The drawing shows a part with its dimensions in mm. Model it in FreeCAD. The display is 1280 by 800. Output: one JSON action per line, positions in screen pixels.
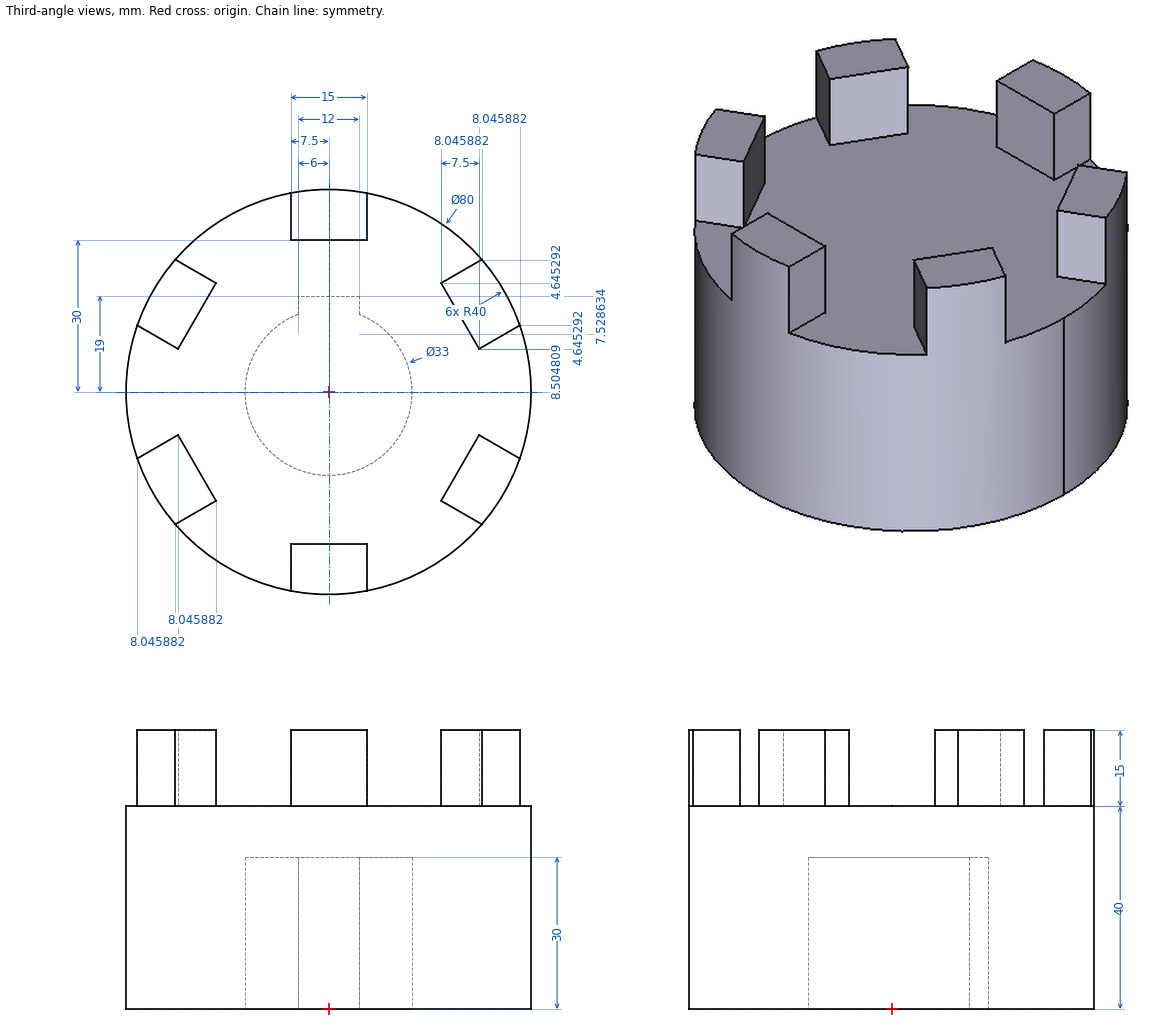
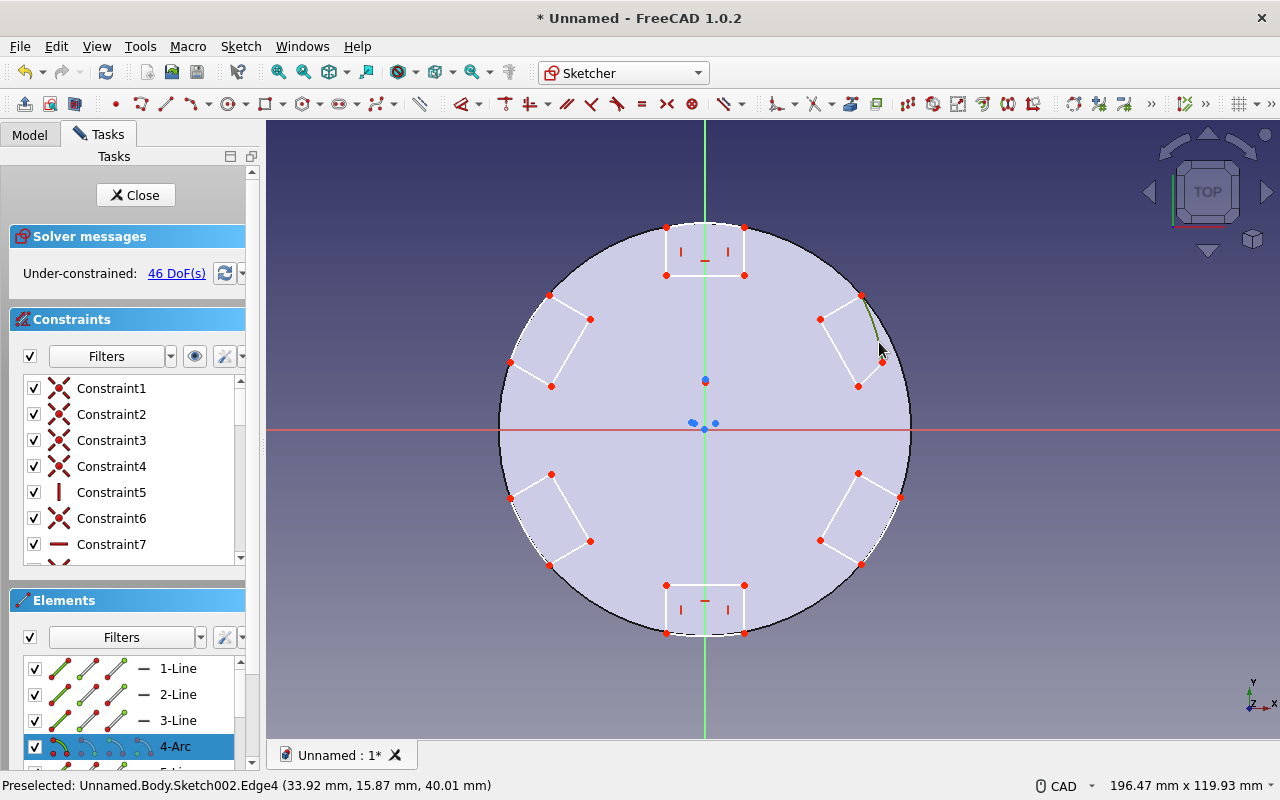
{"action": "left_click", "coordinate": [875, 546]}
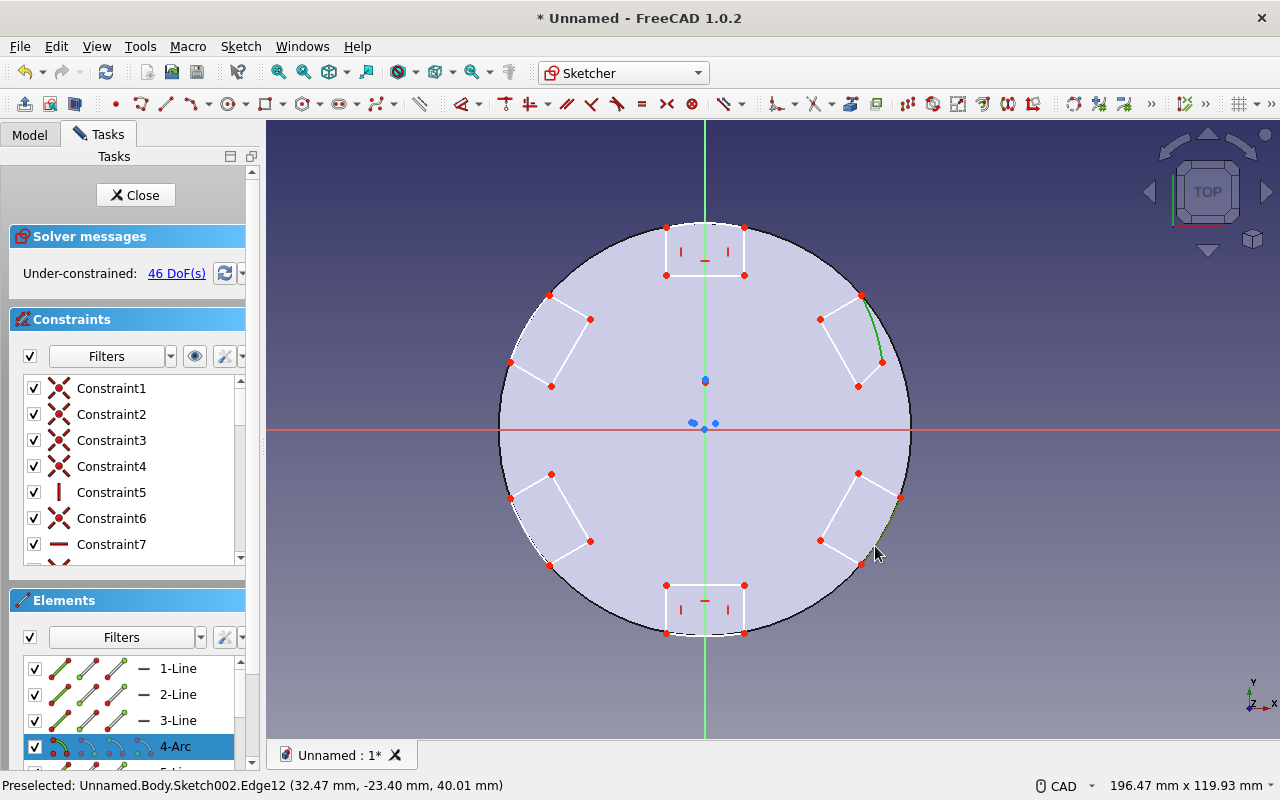
{"action": "key", "text": "c"}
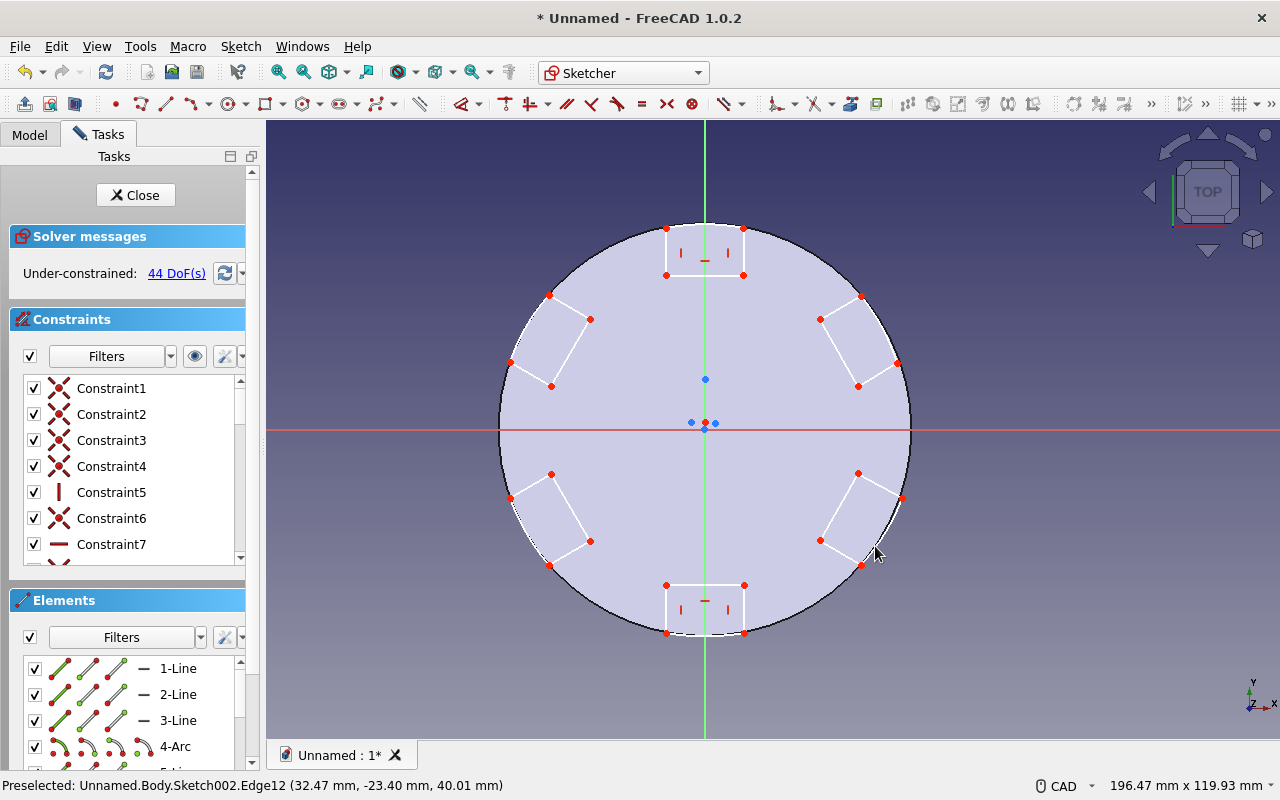
{"action": "left_click", "coordinate": [889, 342]}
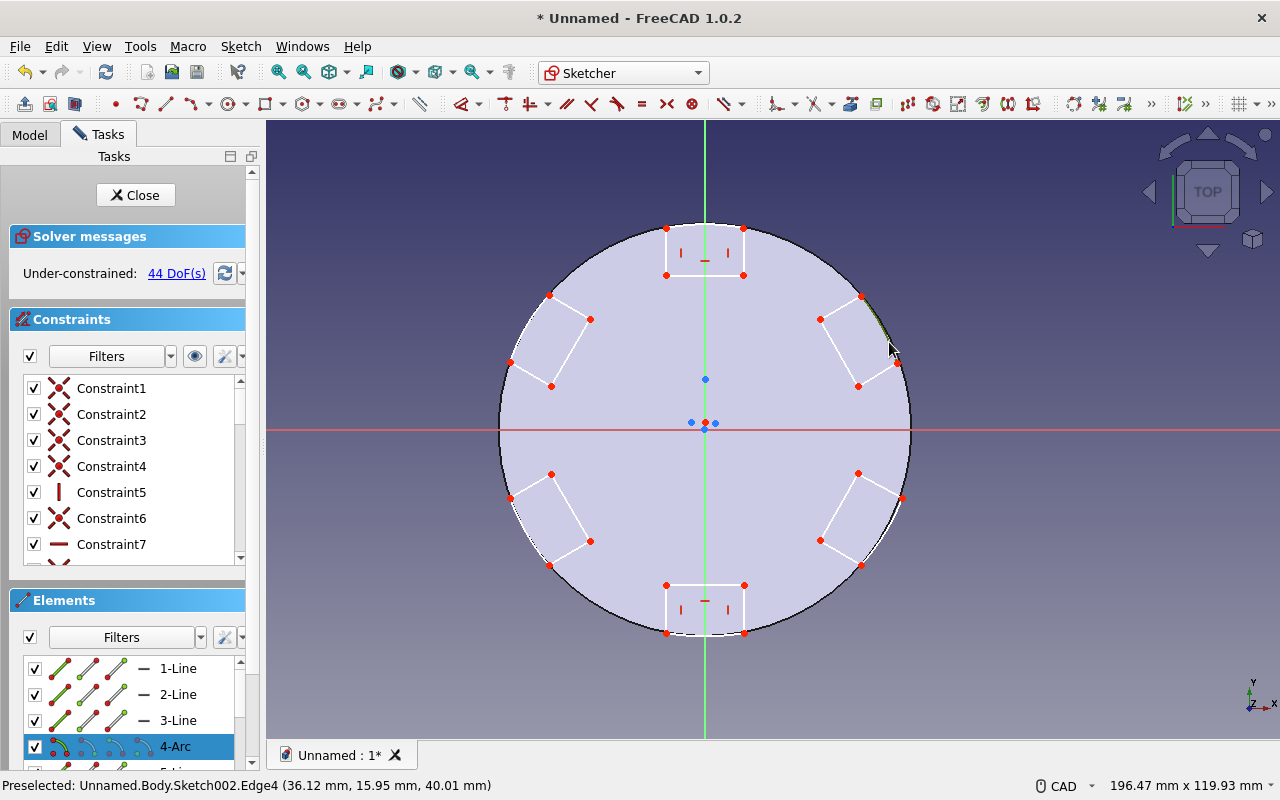
{"action": "left_click", "coordinate": [689, 636]}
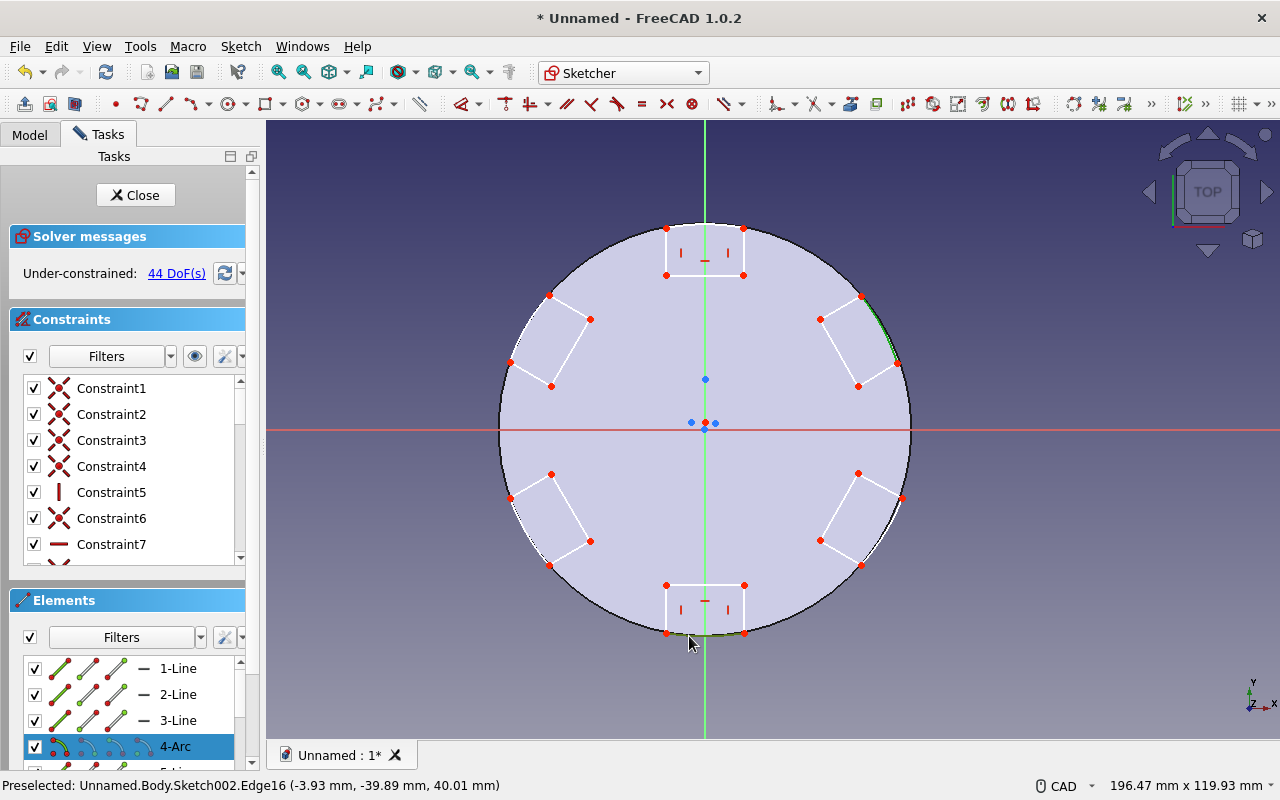
{"action": "key", "text": "c"}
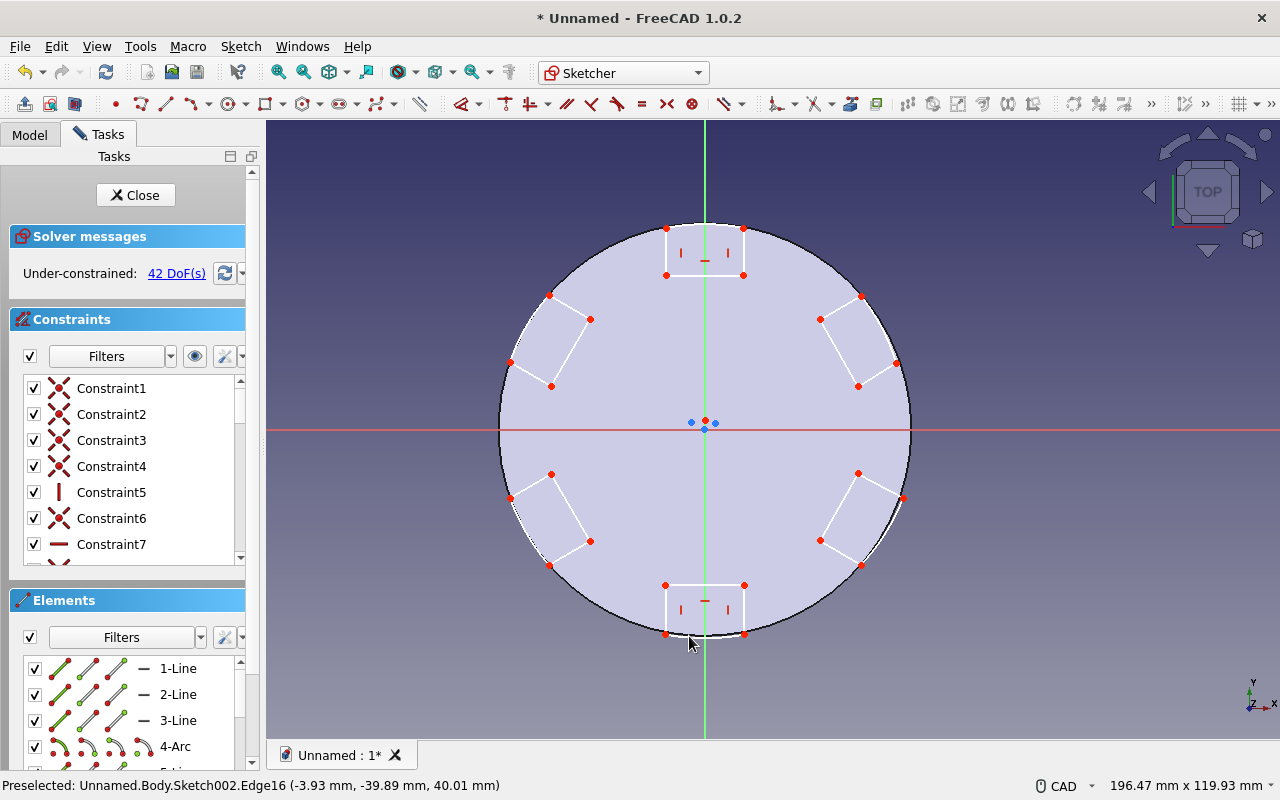
{"action": "left_click", "coordinate": [888, 342]}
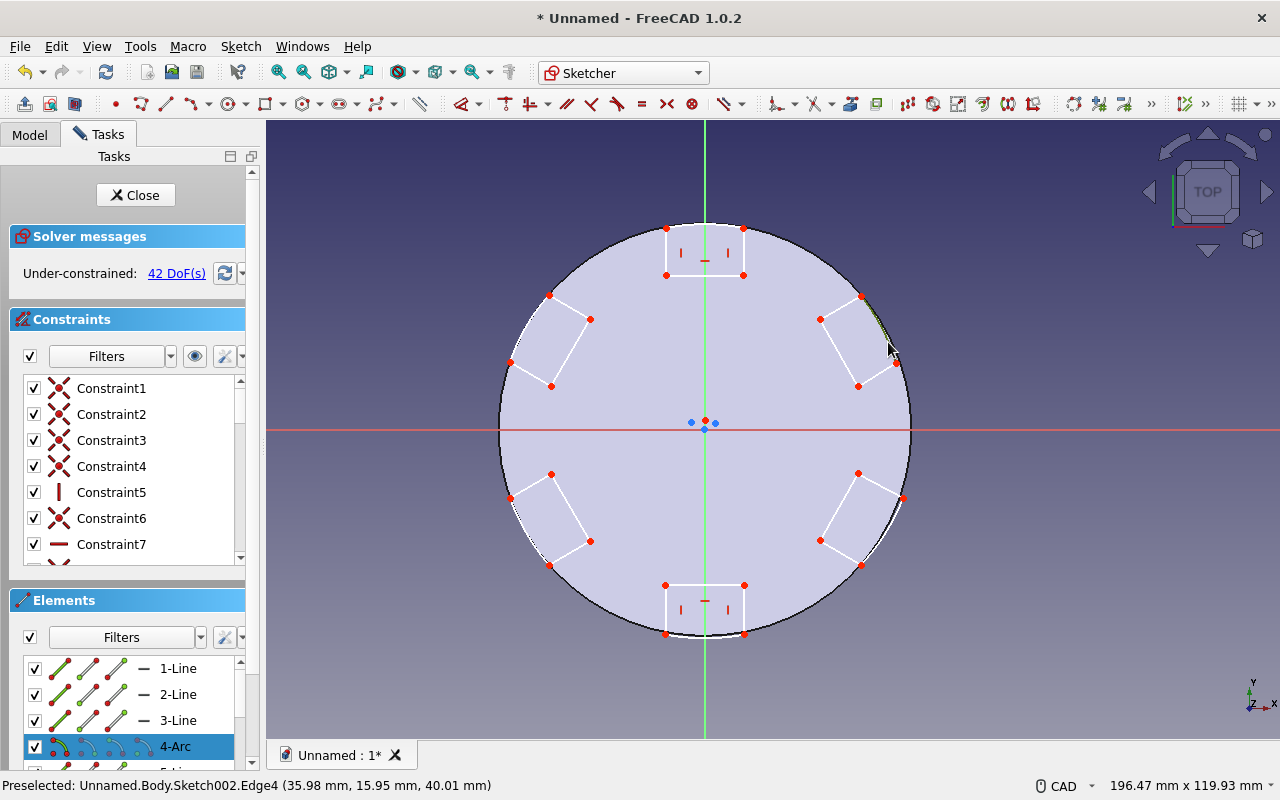
{"action": "left_click", "coordinate": [519, 520]}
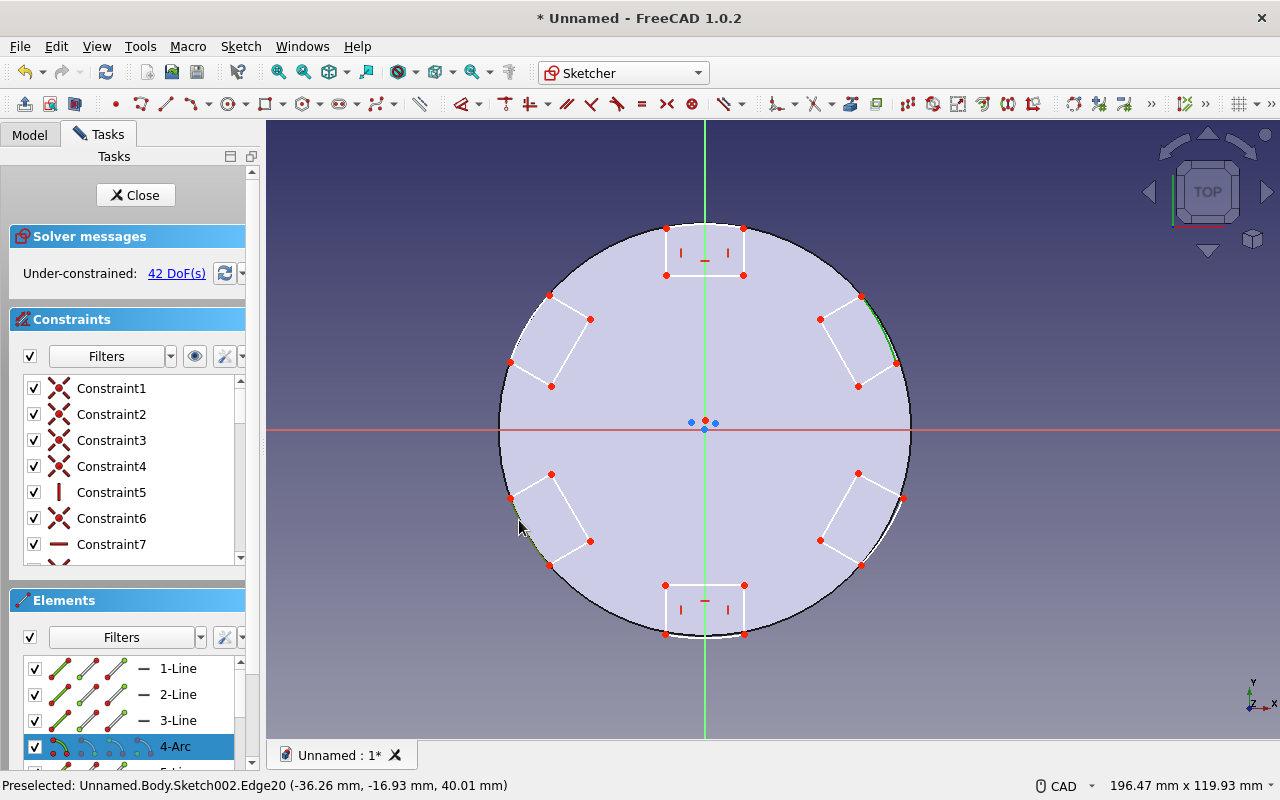
{"action": "key", "text": "c"}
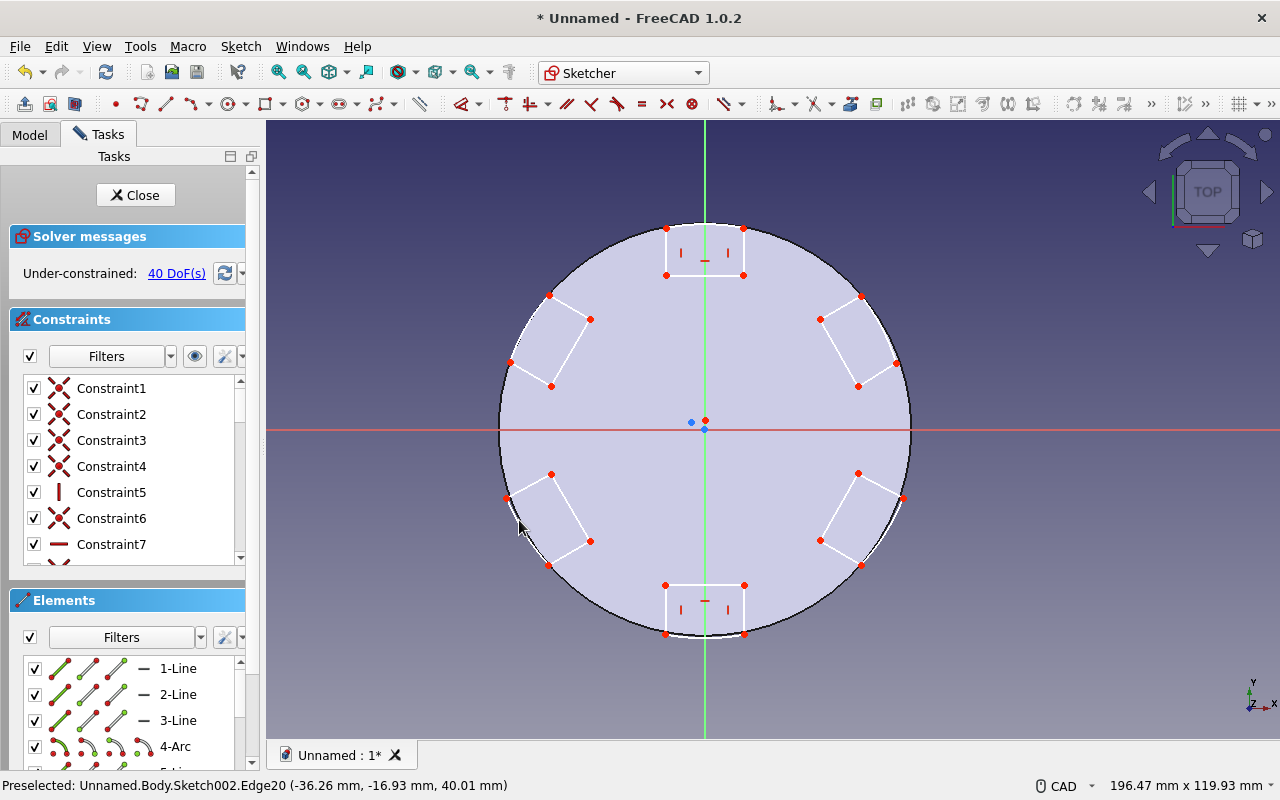
{"action": "left_click", "coordinate": [888, 342]}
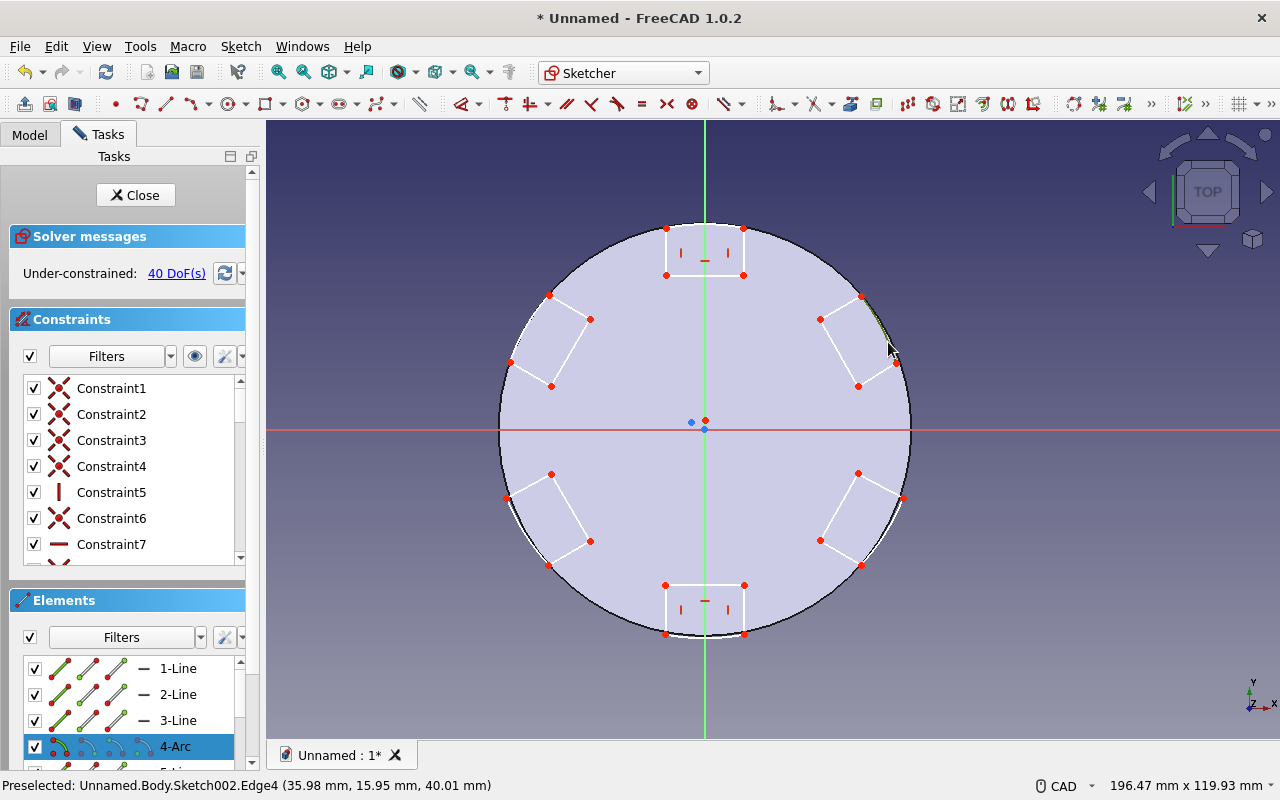
{"action": "left_click", "coordinate": [534, 314]}